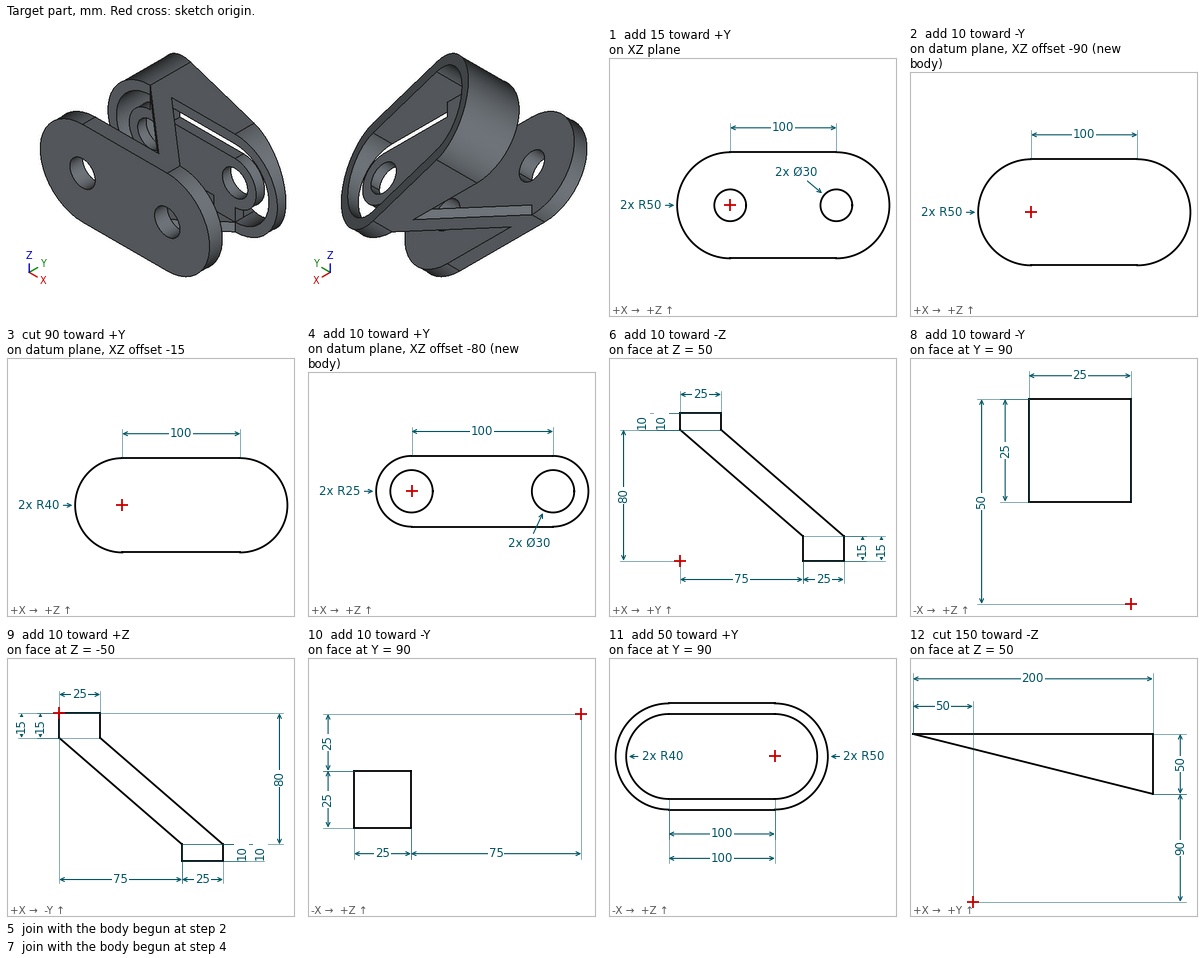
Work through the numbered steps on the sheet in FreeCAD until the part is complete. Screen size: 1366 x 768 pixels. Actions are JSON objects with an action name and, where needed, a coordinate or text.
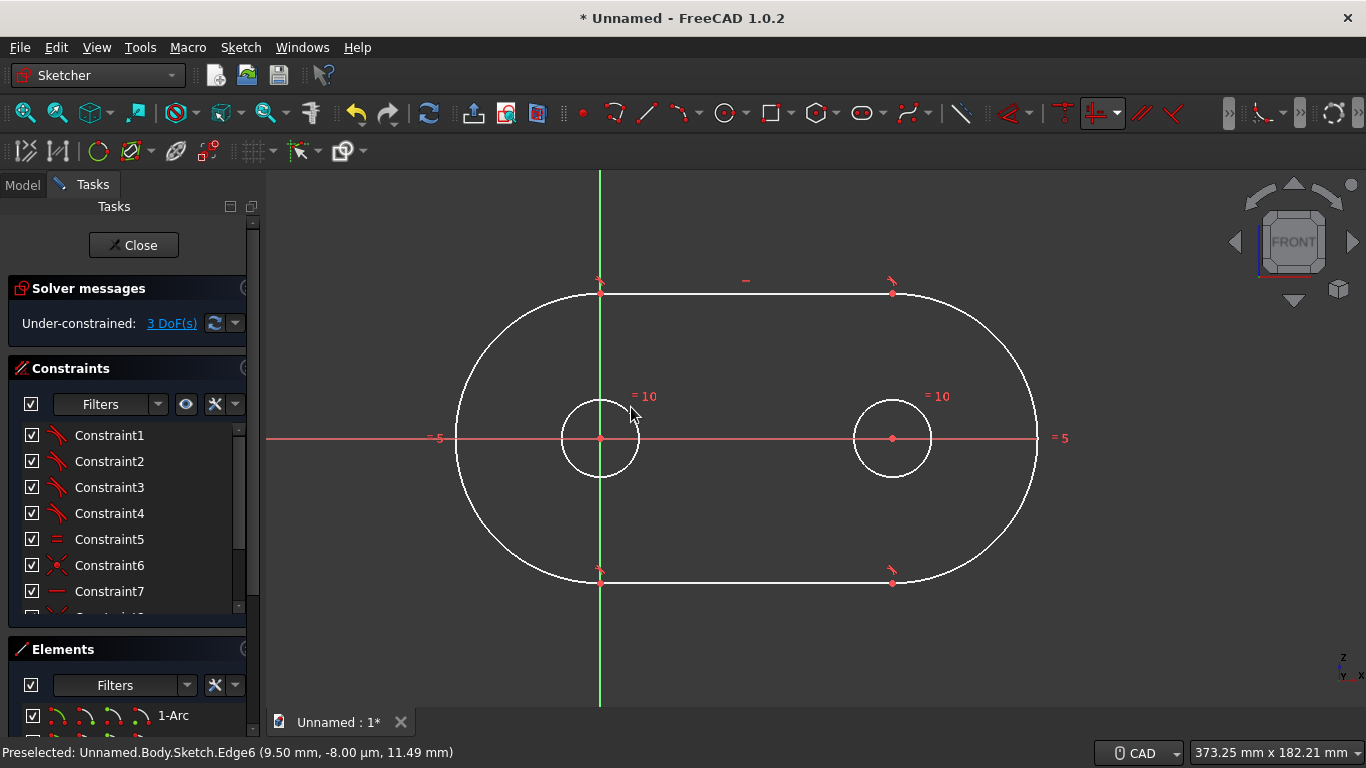
{"action": "left_click", "coordinate": [1008, 114]}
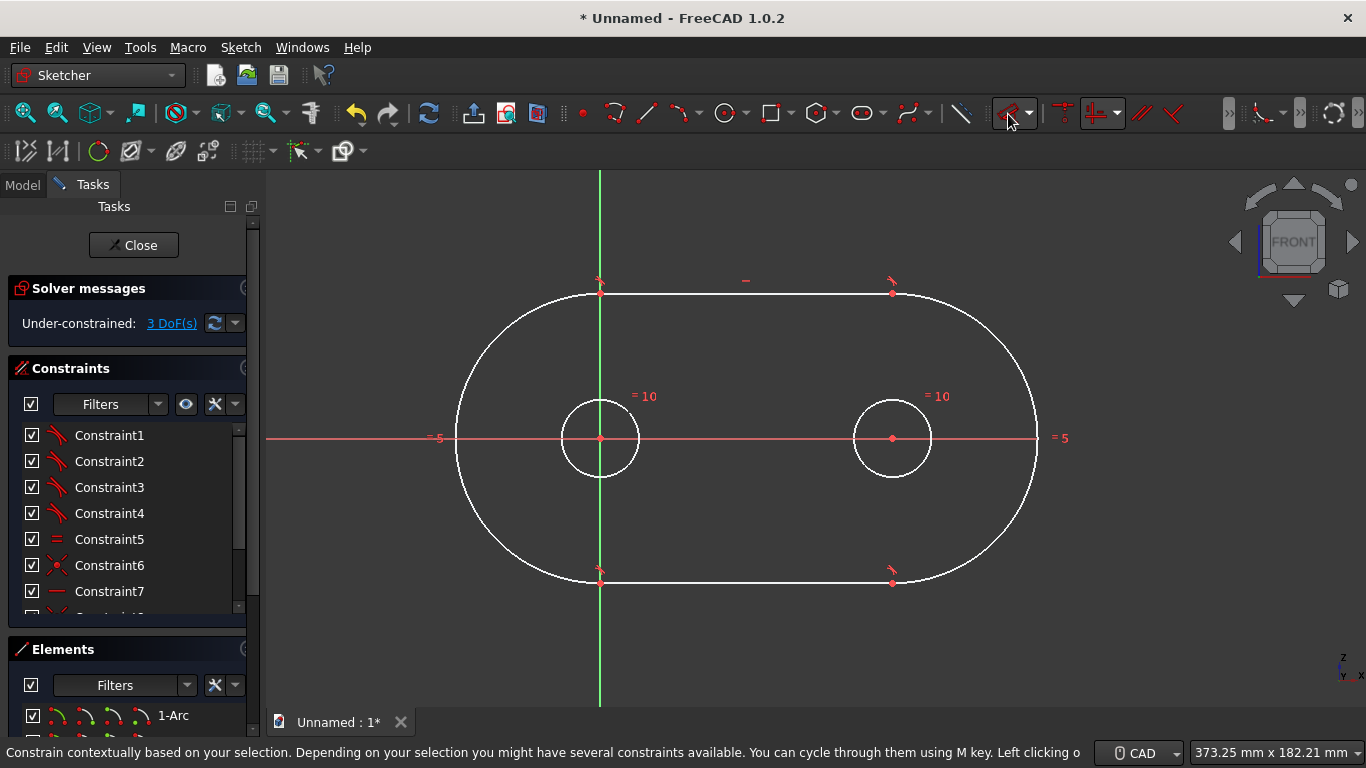
{"action": "left_click", "coordinate": [483, 353]}
{"action": "left_click", "coordinate": [457, 334]}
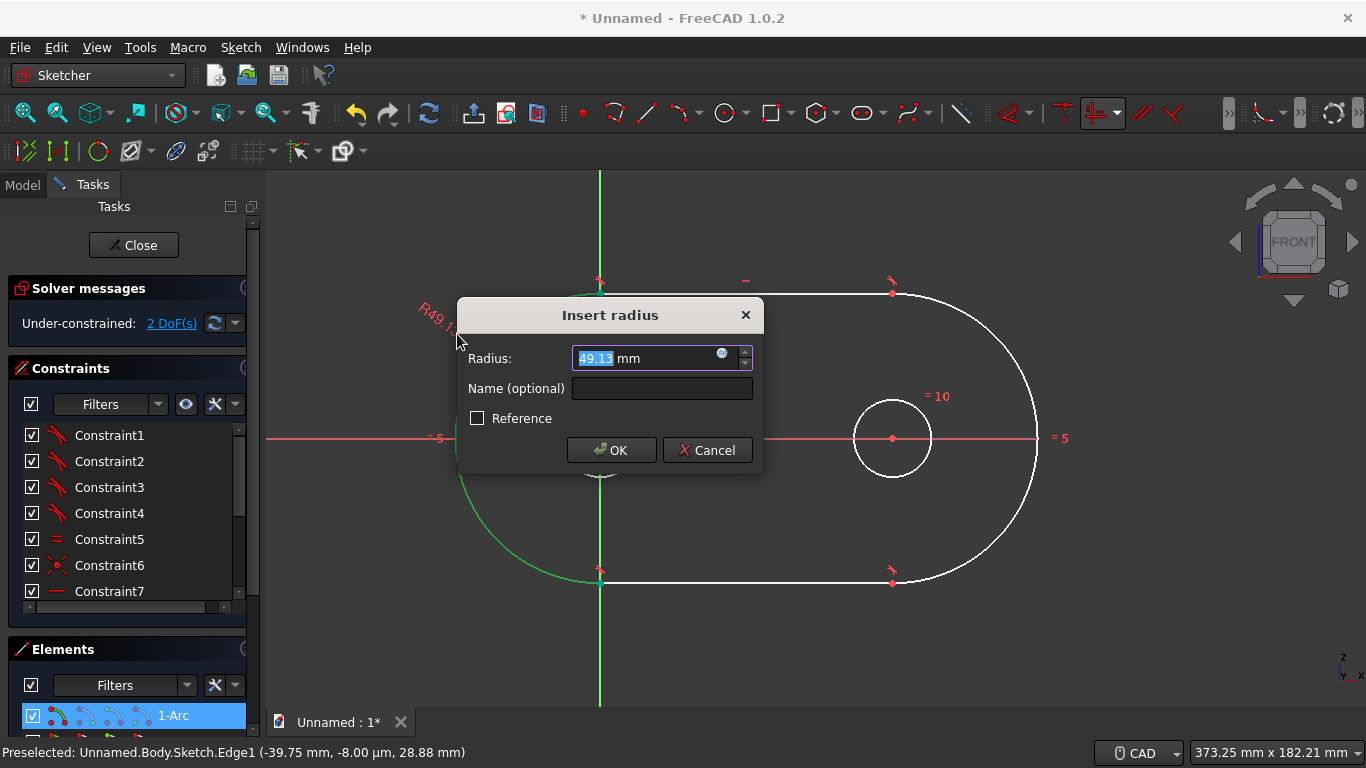
{"action": "type", "text": "50"}
{"action": "key", "text": "Return"}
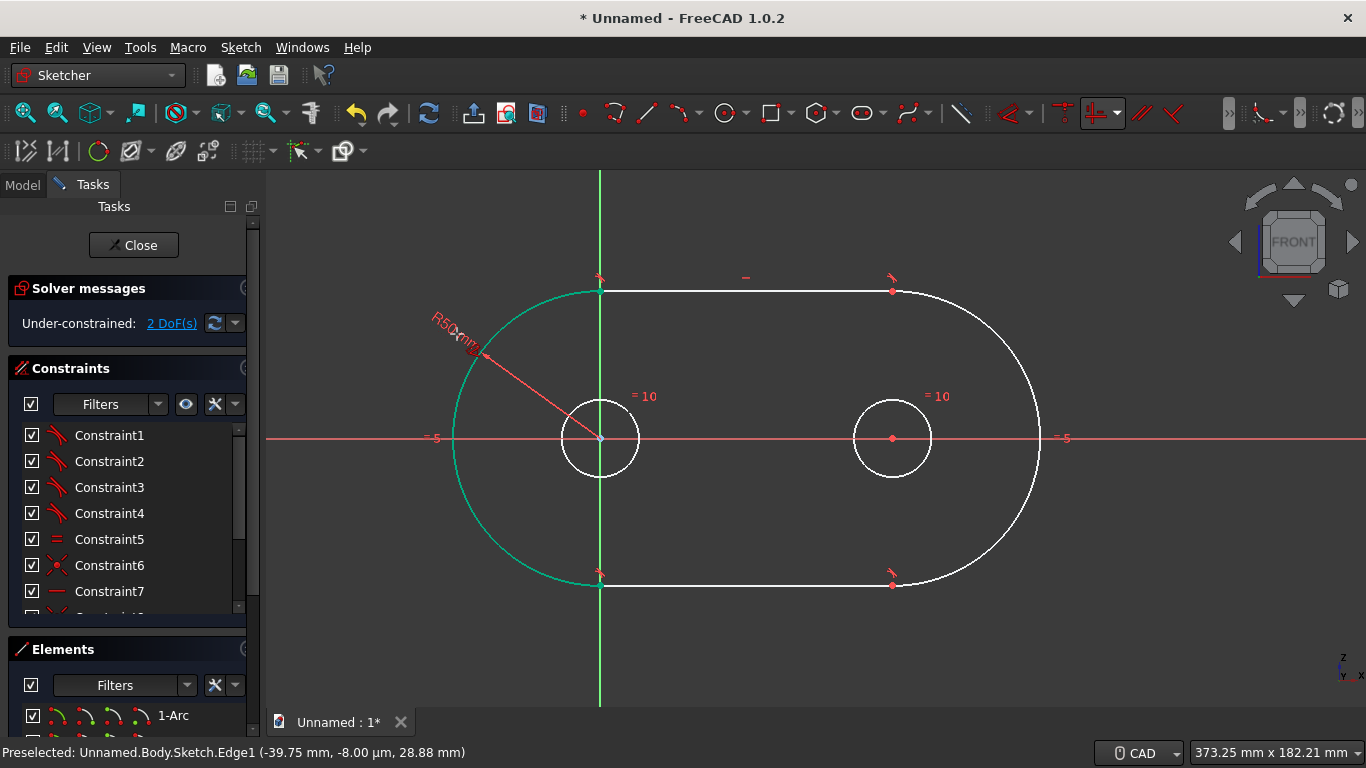
{"action": "left_click", "coordinate": [920, 411]}
{"action": "left_click", "coordinate": [943, 388]}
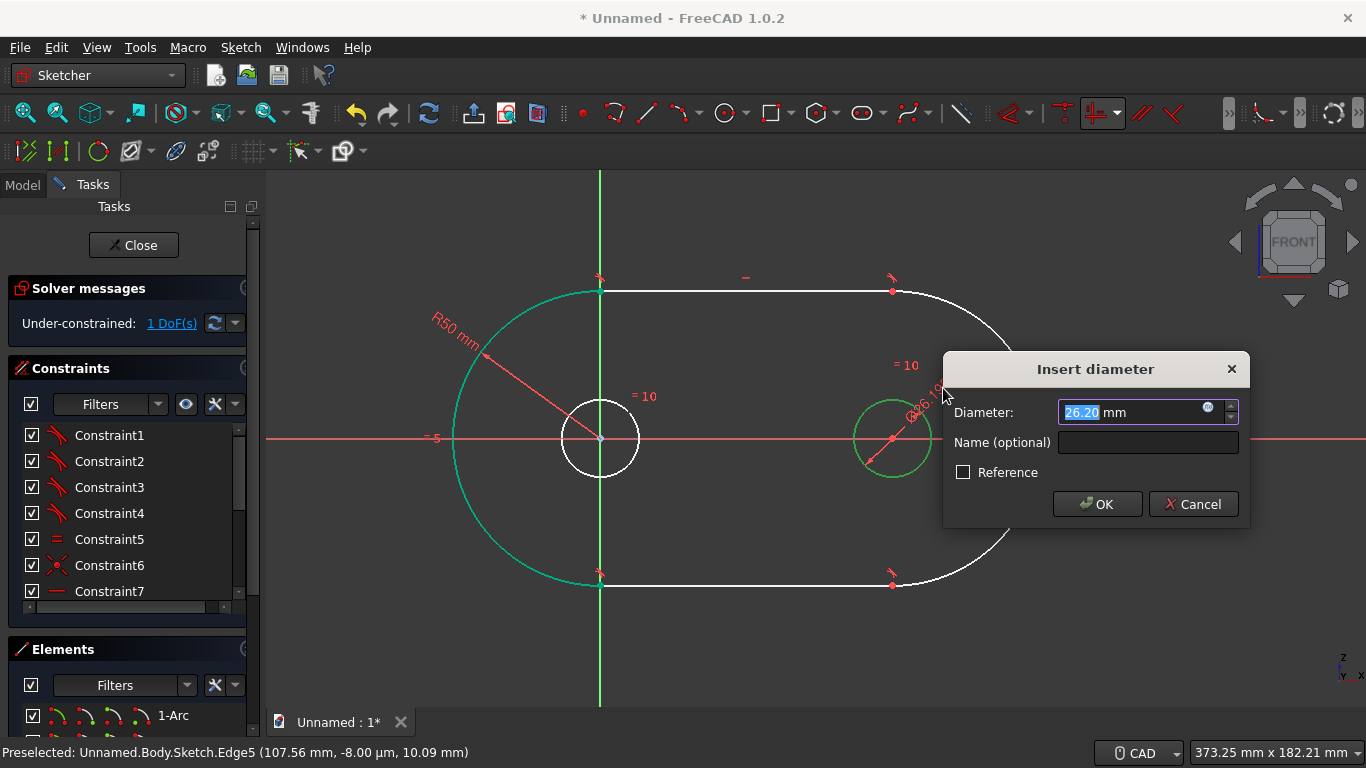
{"action": "type", "text": "30"}
{"action": "key", "text": "Return"}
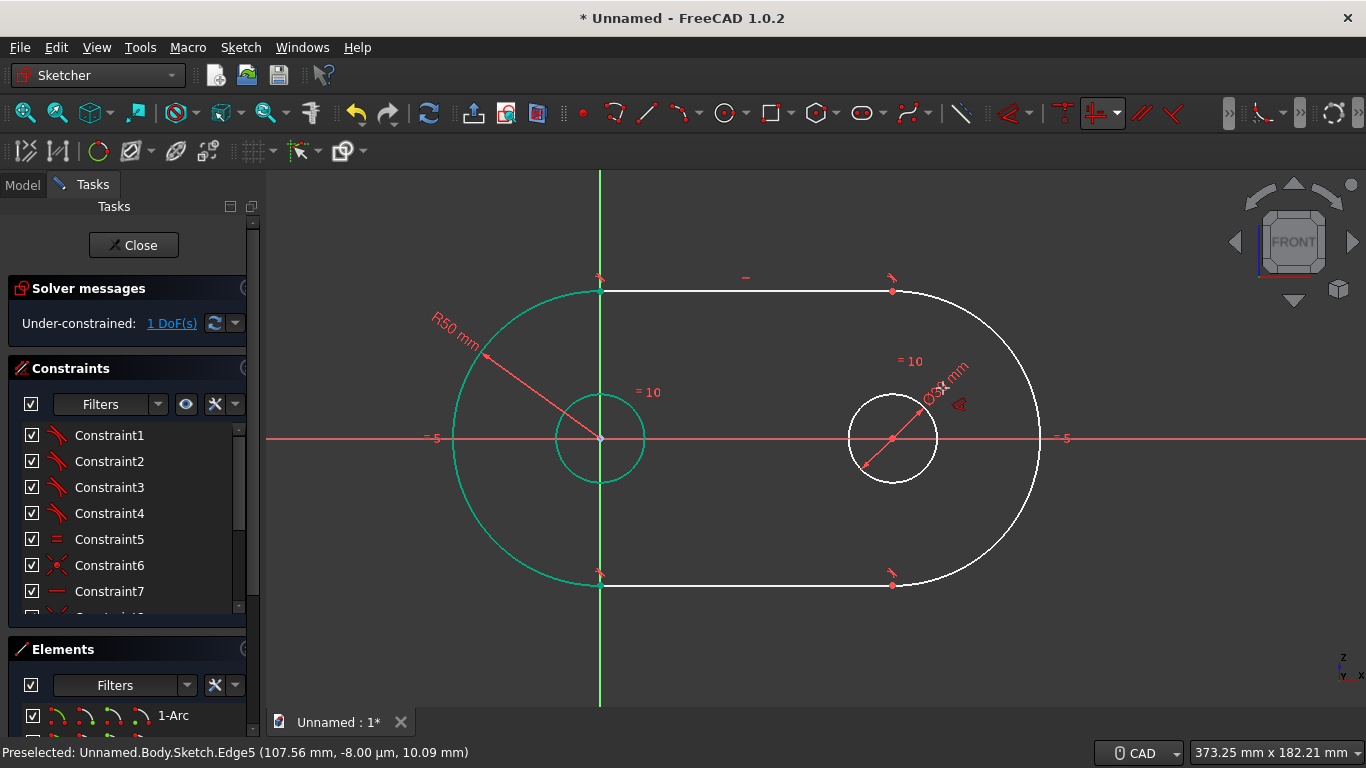
{"action": "left_click", "coordinate": [688, 291]}
{"action": "left_click", "coordinate": [747, 257]}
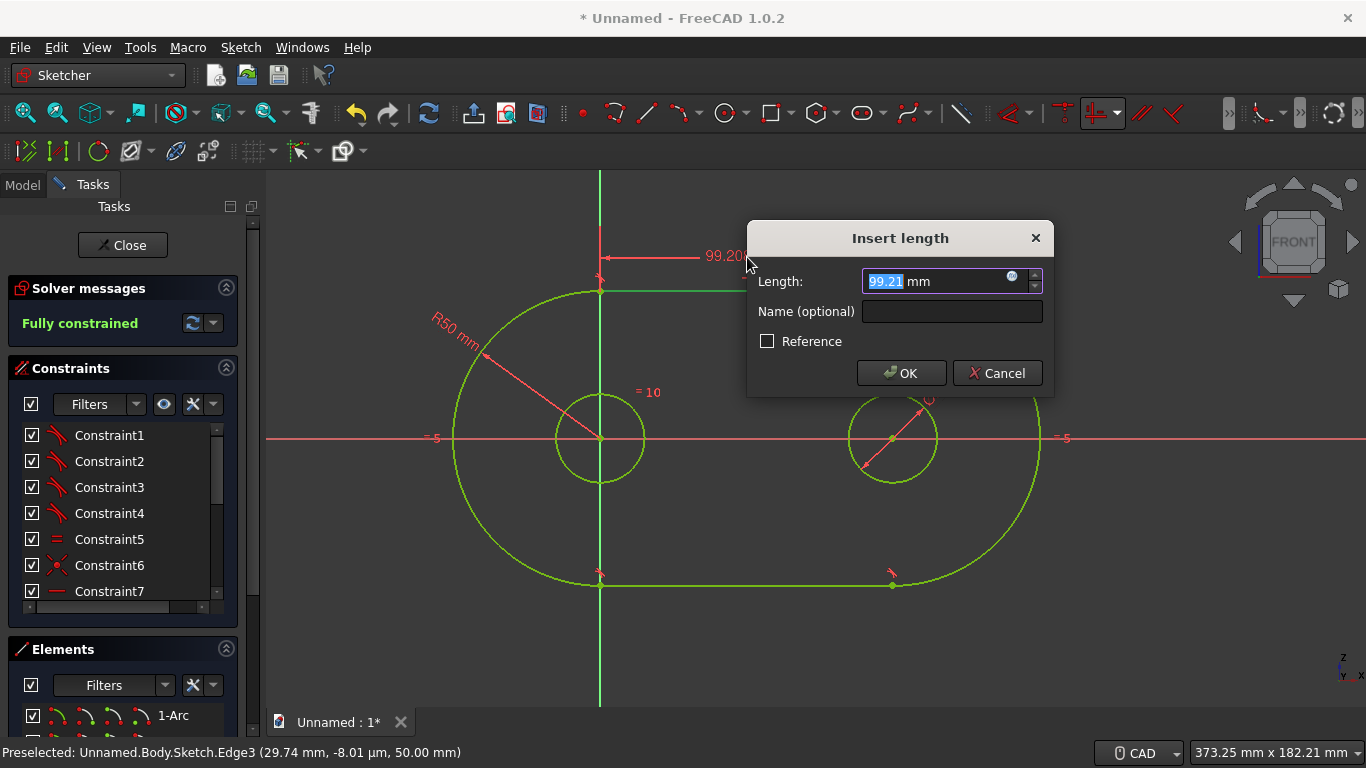
{"action": "type", "text": "100"}
{"action": "key", "text": "Return"}
{"action": "key", "text": "Escape"}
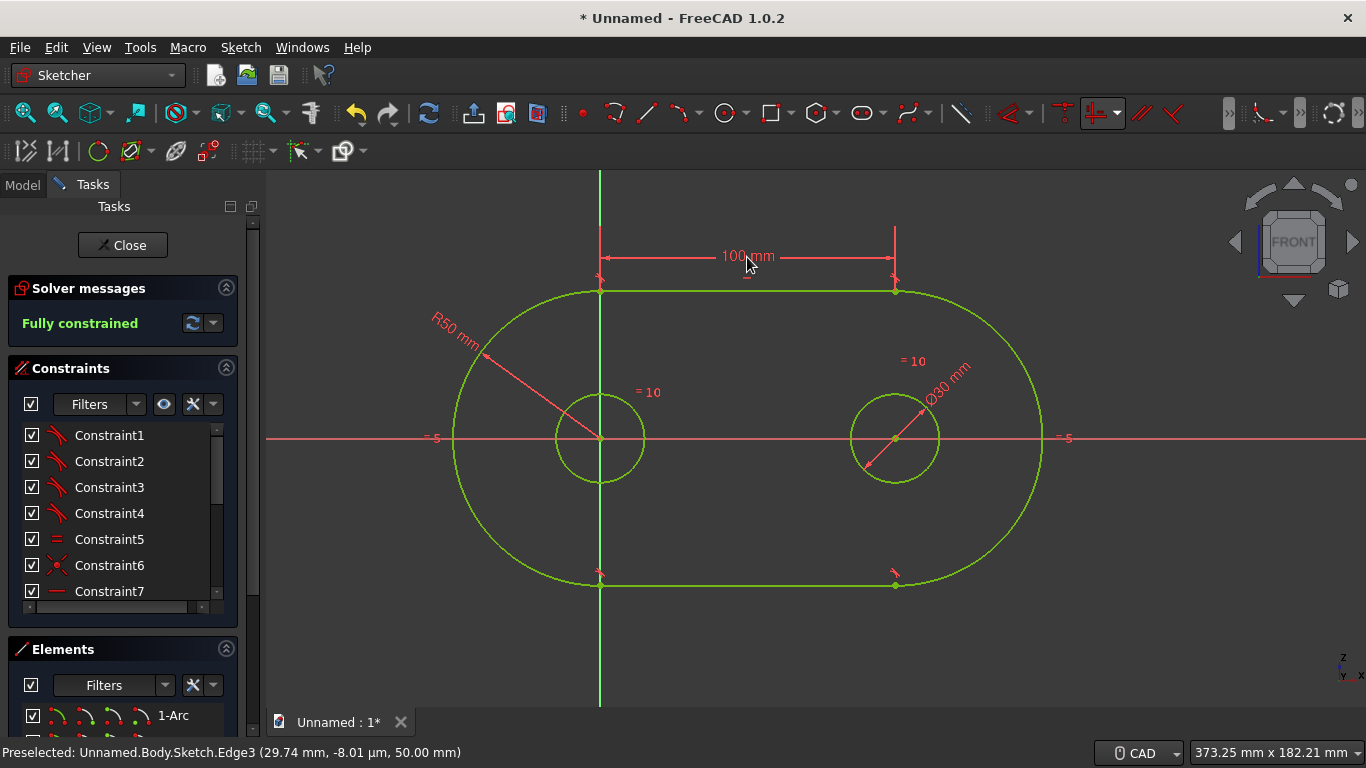
{"action": "left_click", "coordinate": [123, 245]}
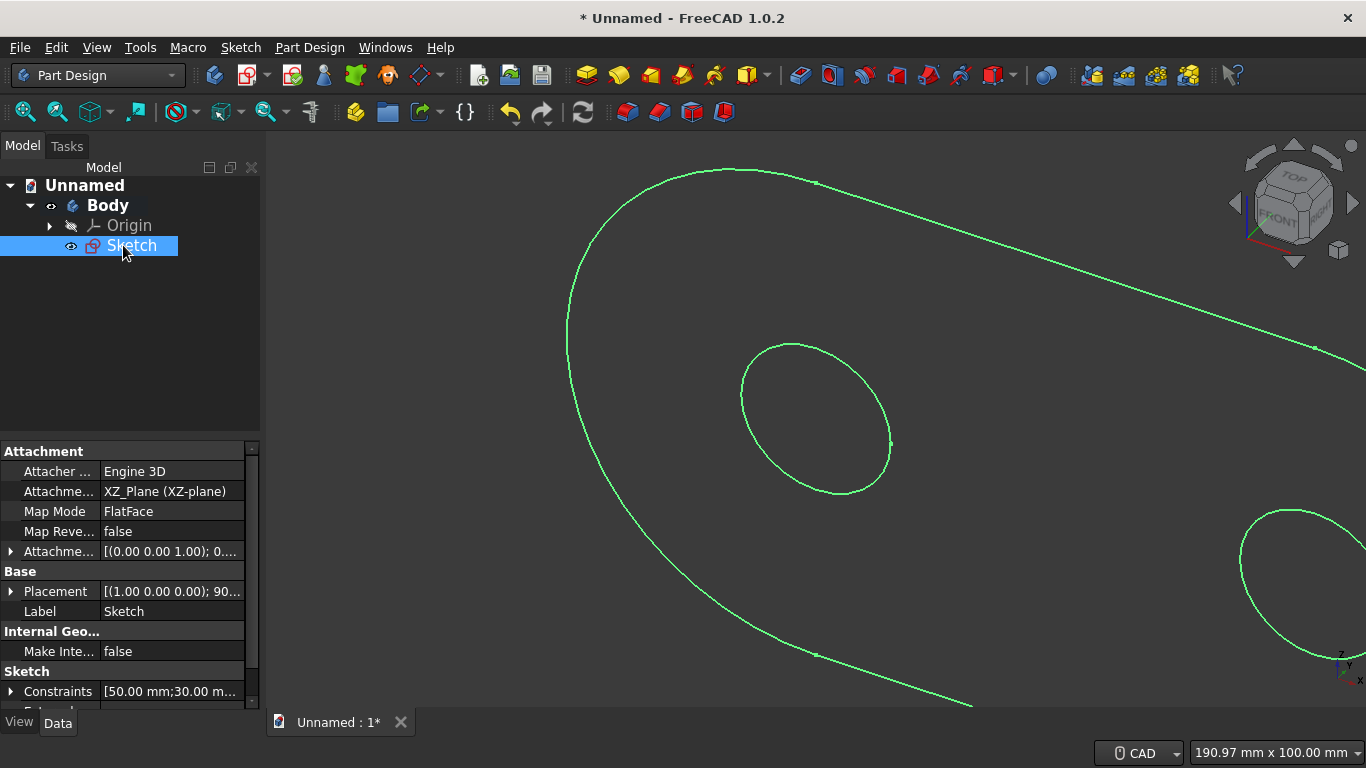
{"action": "left_click", "coordinate": [588, 76]}